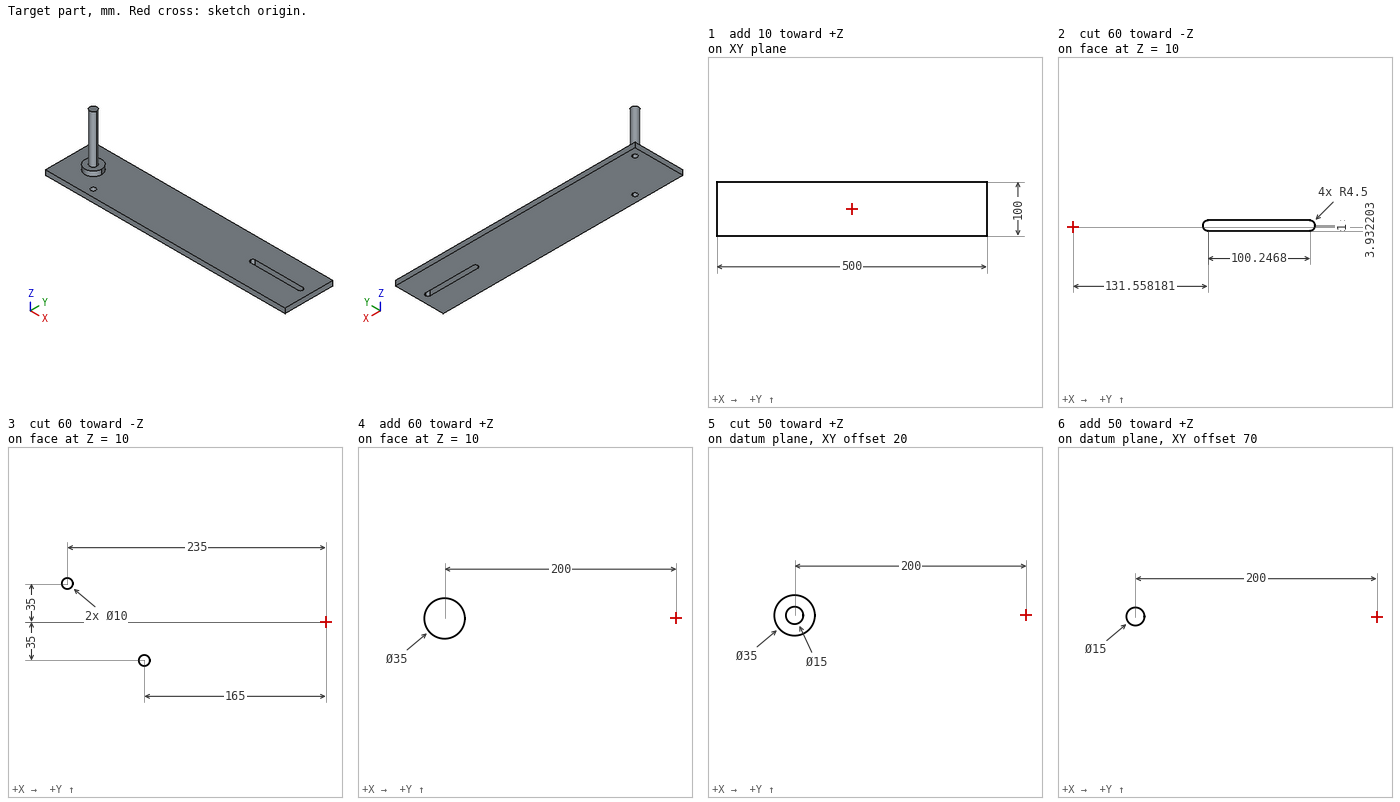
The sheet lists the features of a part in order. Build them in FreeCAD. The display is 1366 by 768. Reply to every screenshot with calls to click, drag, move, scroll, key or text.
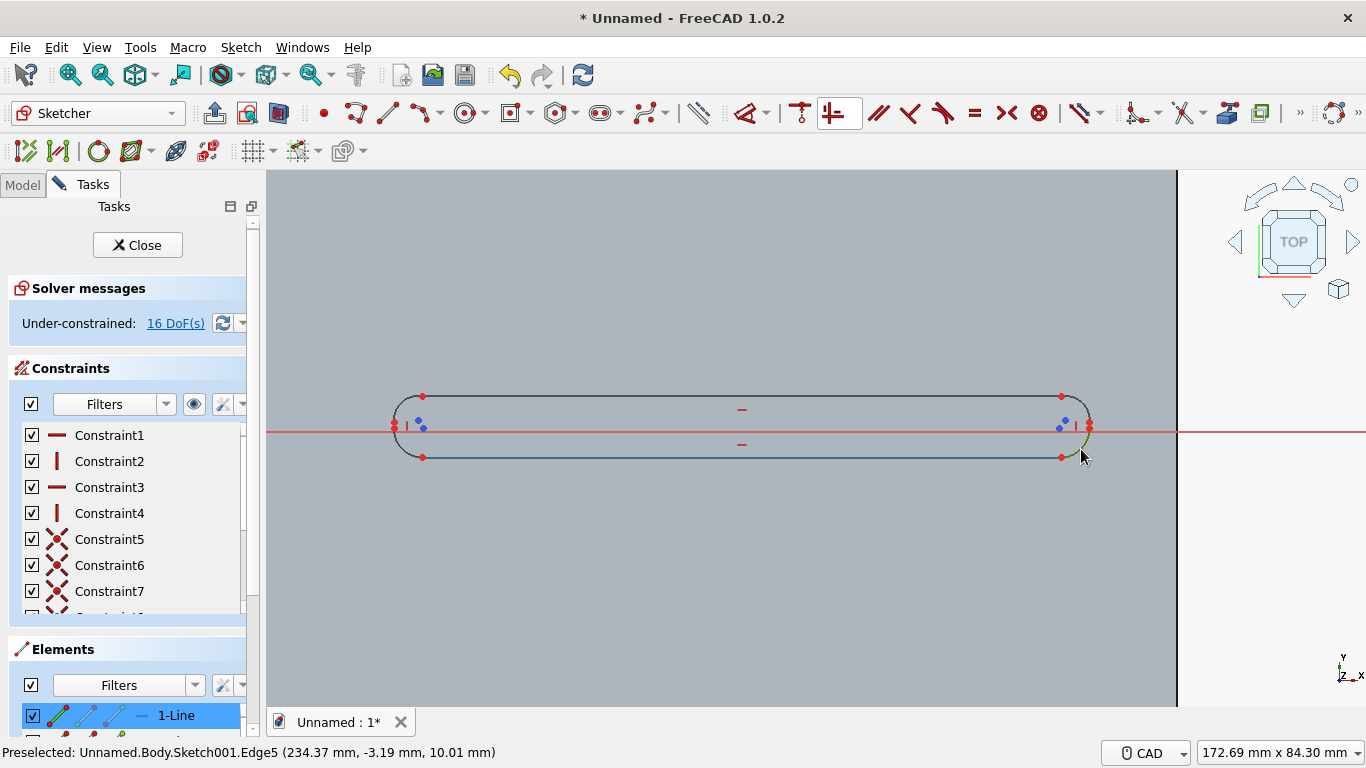
key(t)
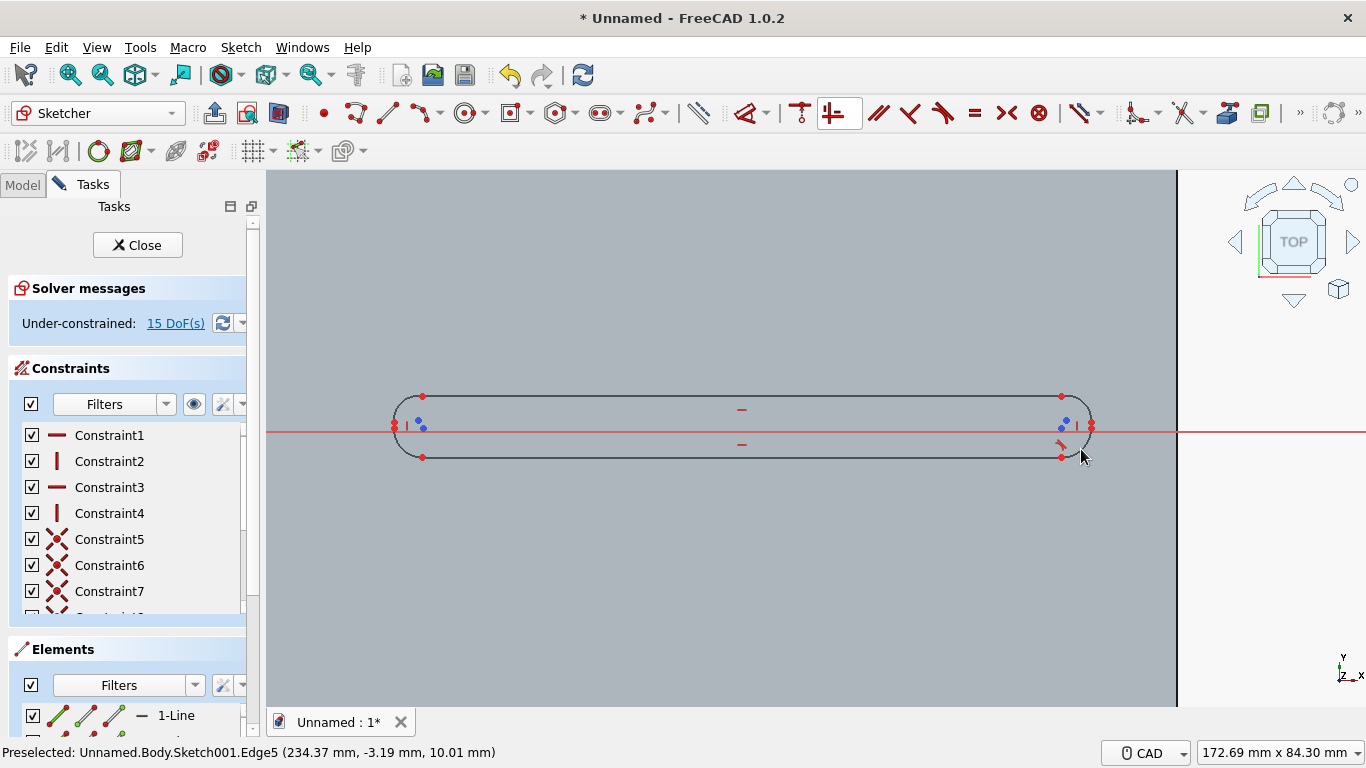
click(614, 458)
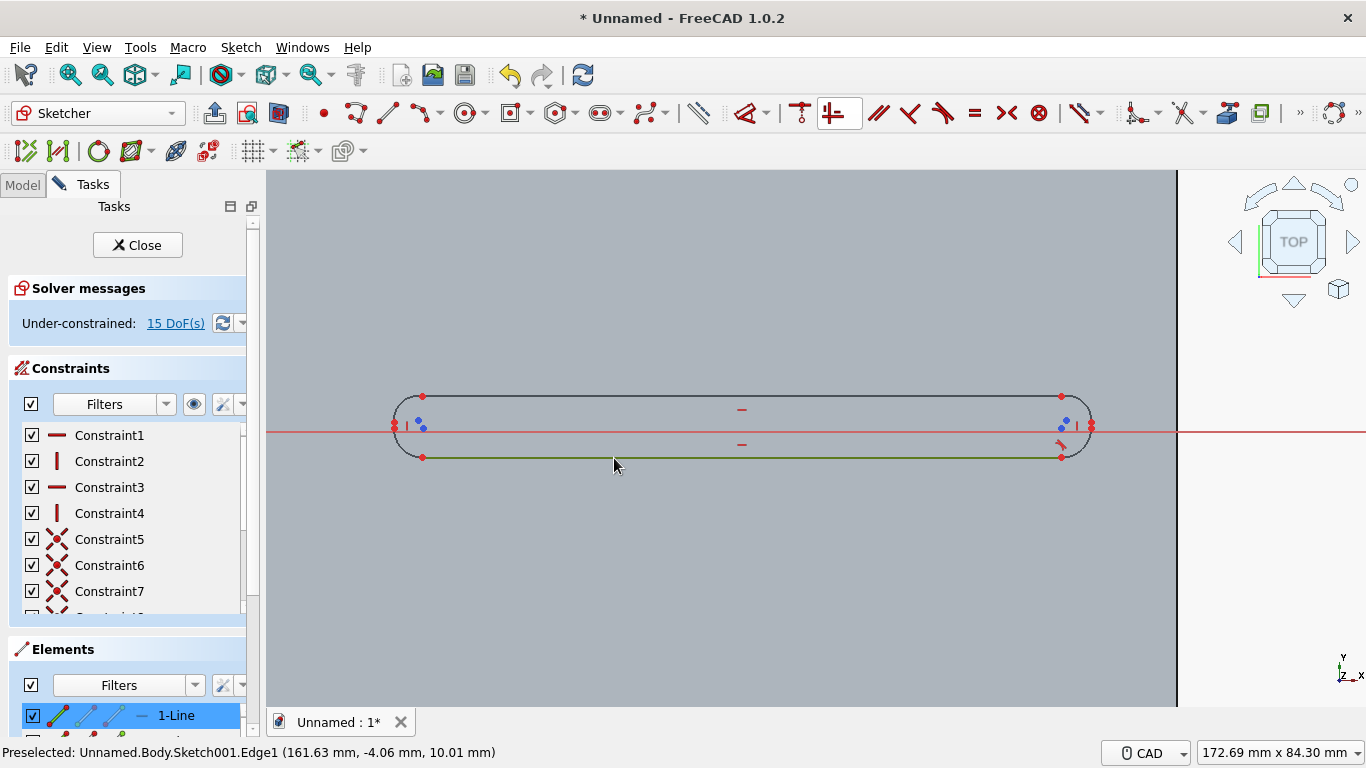
scroll(397, 442, up, 2)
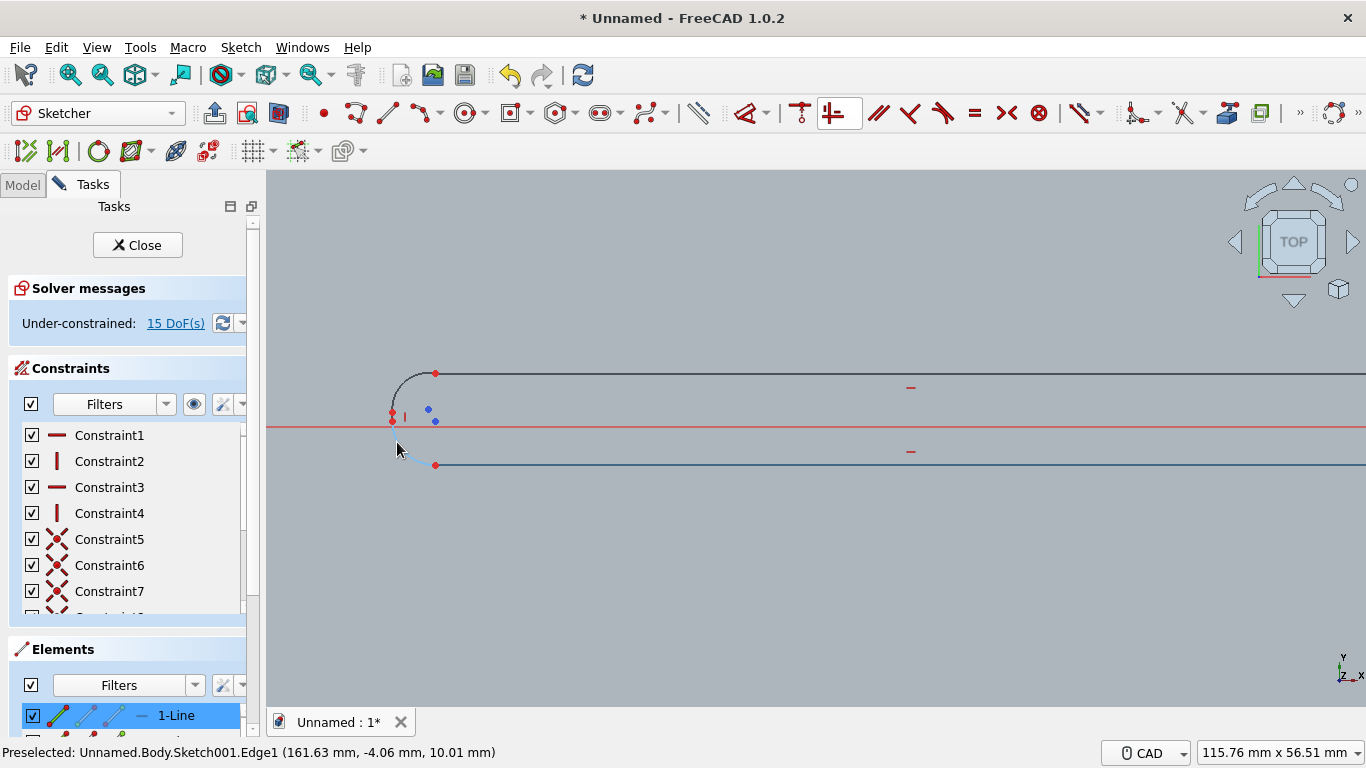
click(397, 441)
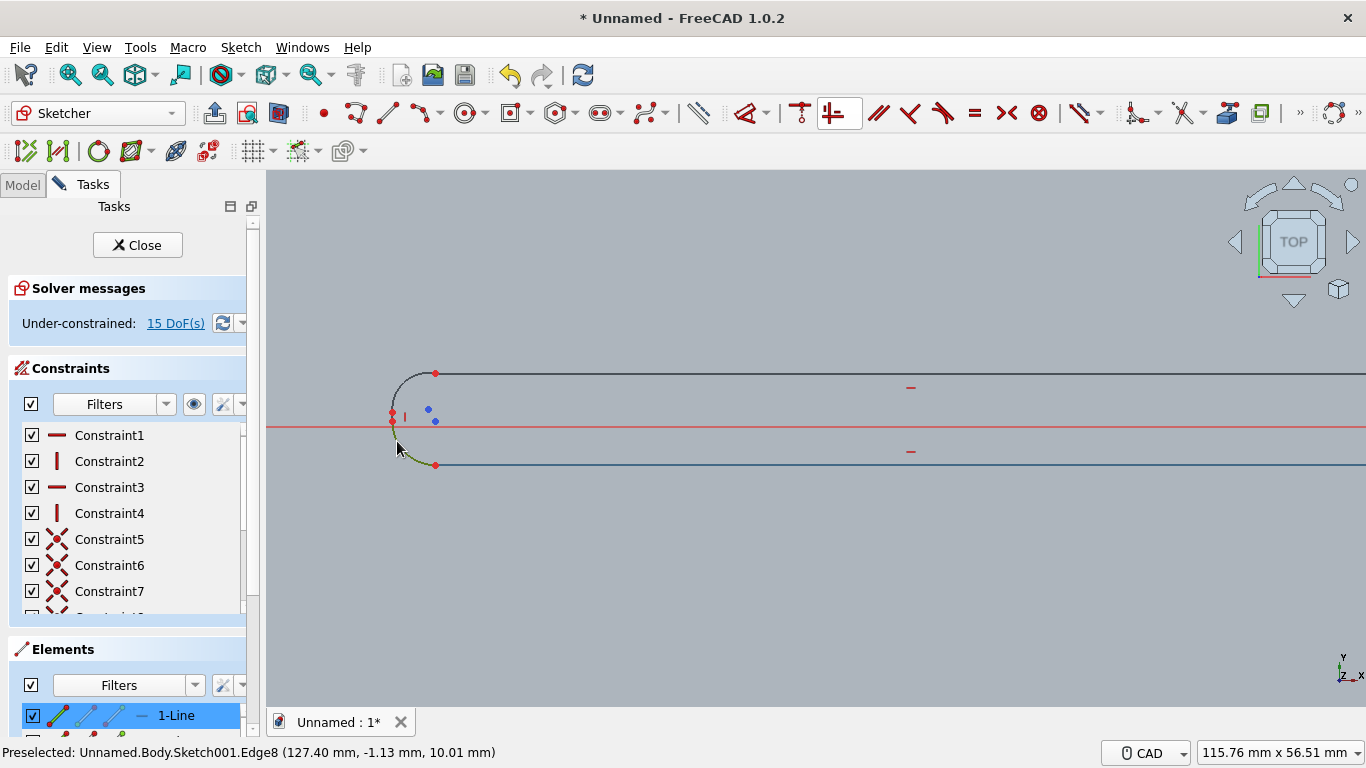
click(944, 114)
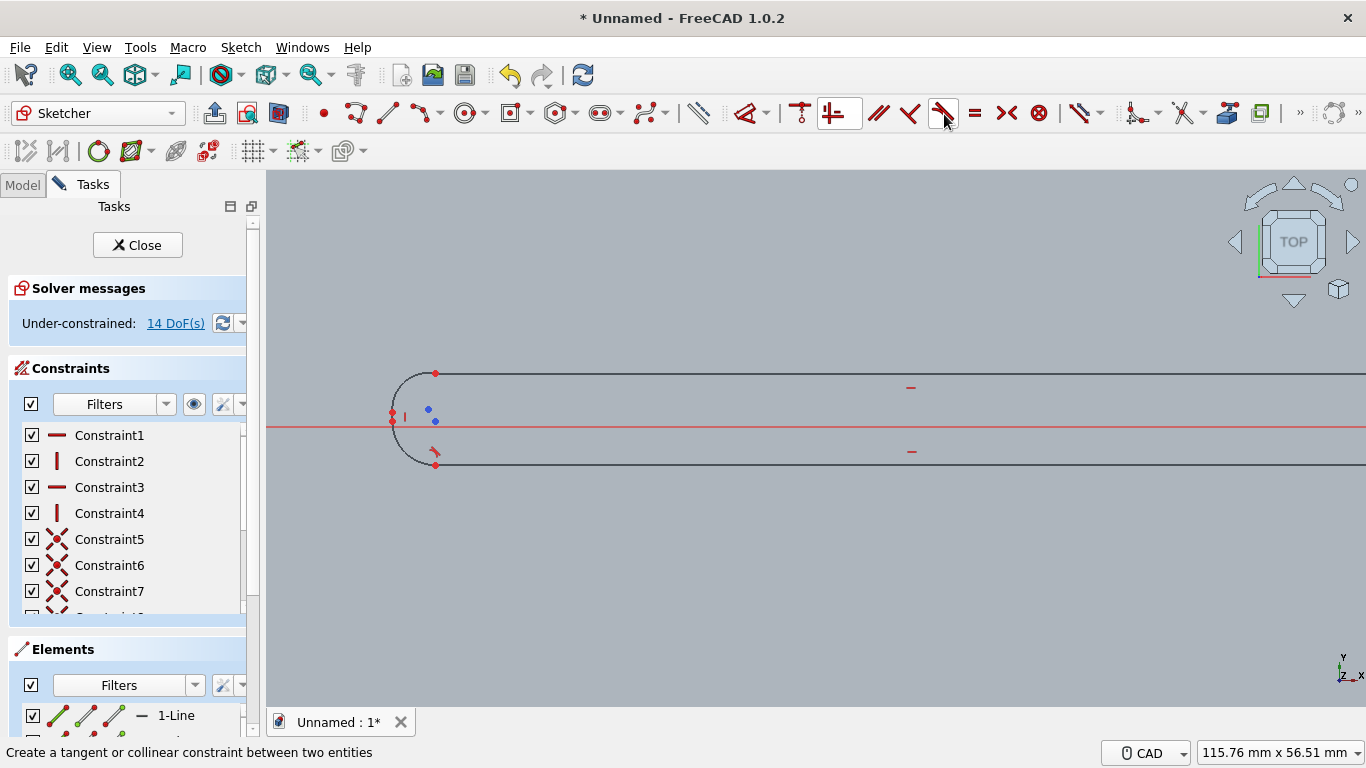
scroll(937, 448, down, 6)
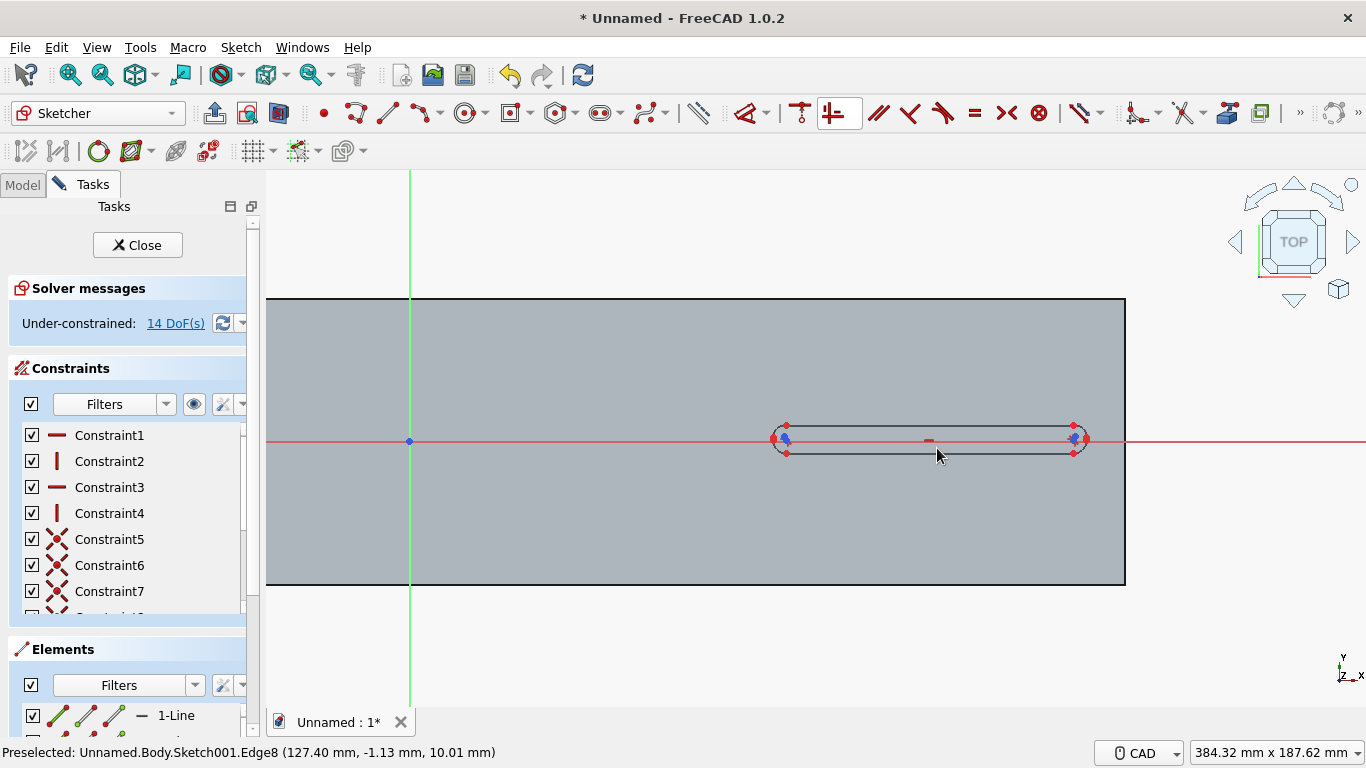
scroll(1087, 439, up, 12)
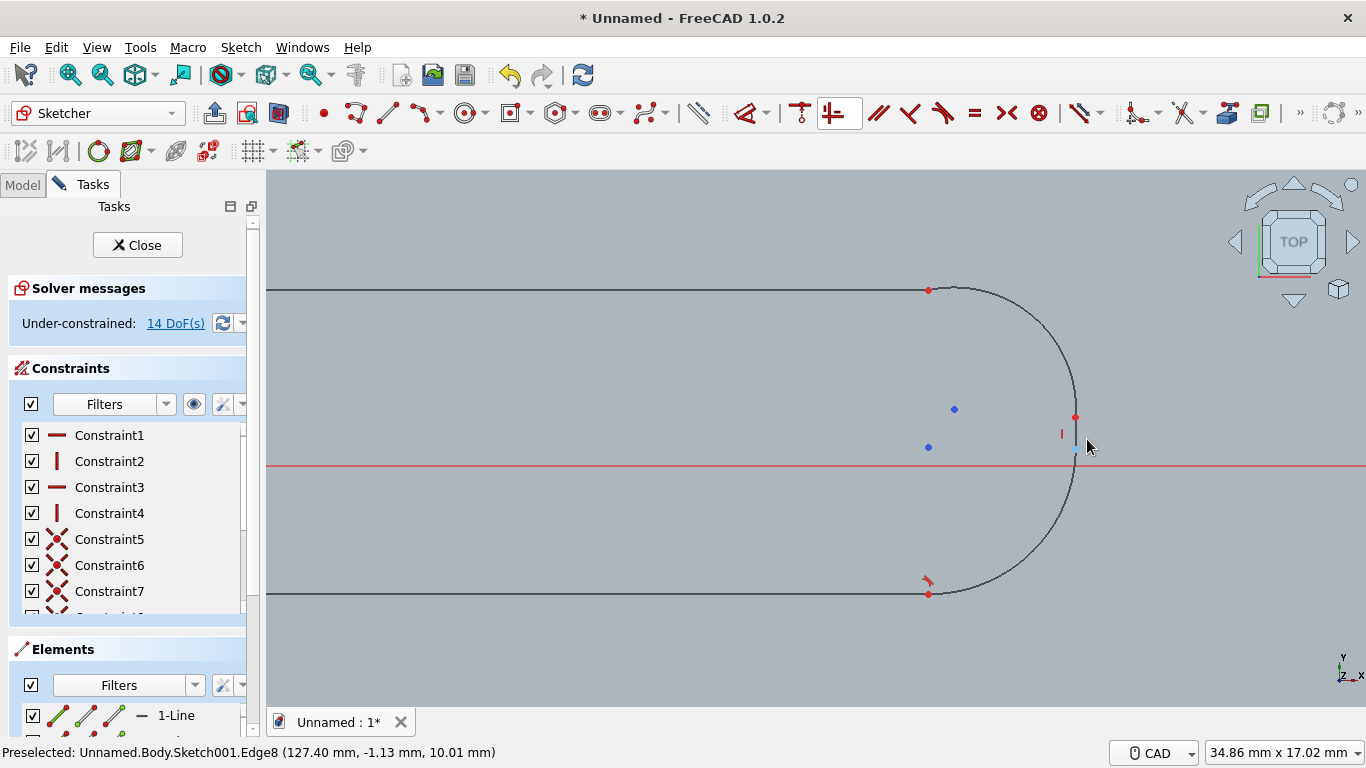
click(1076, 434)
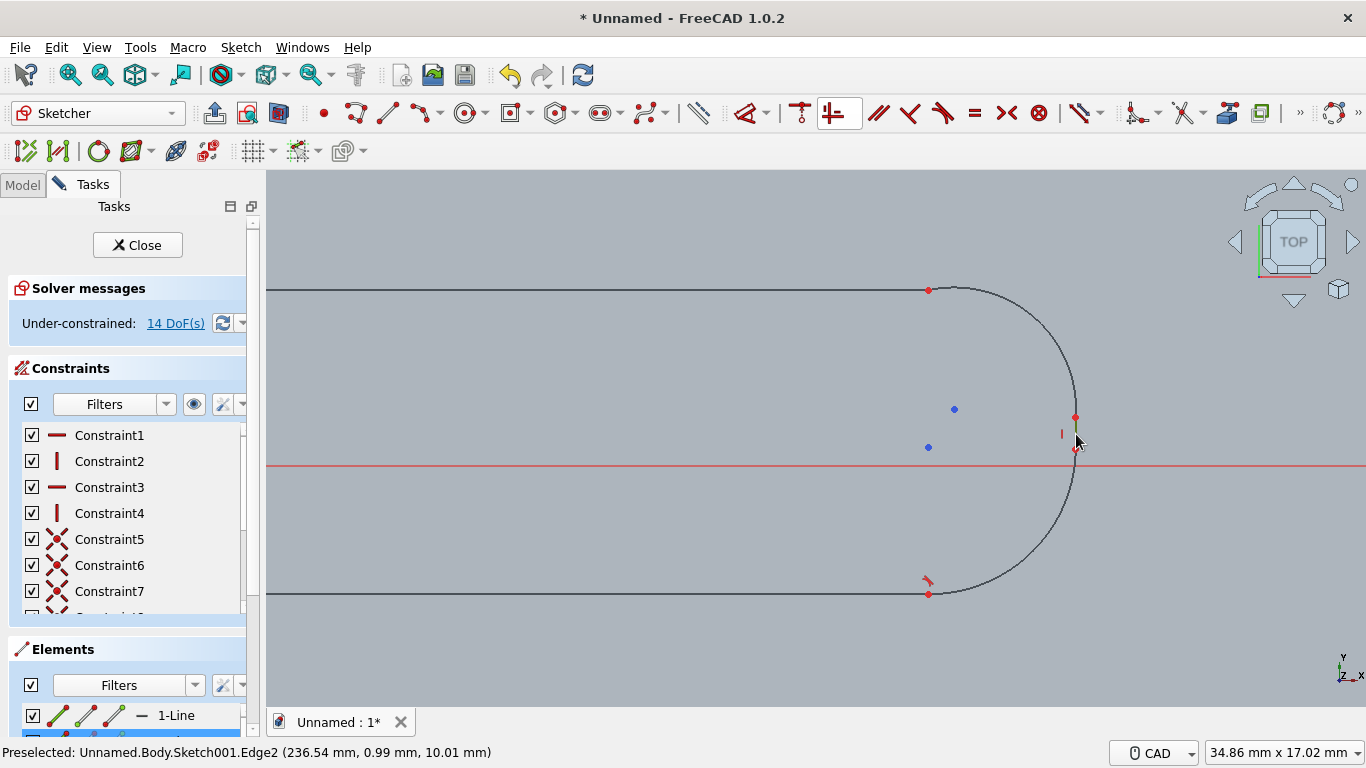
scroll(1087, 439, down, 12)